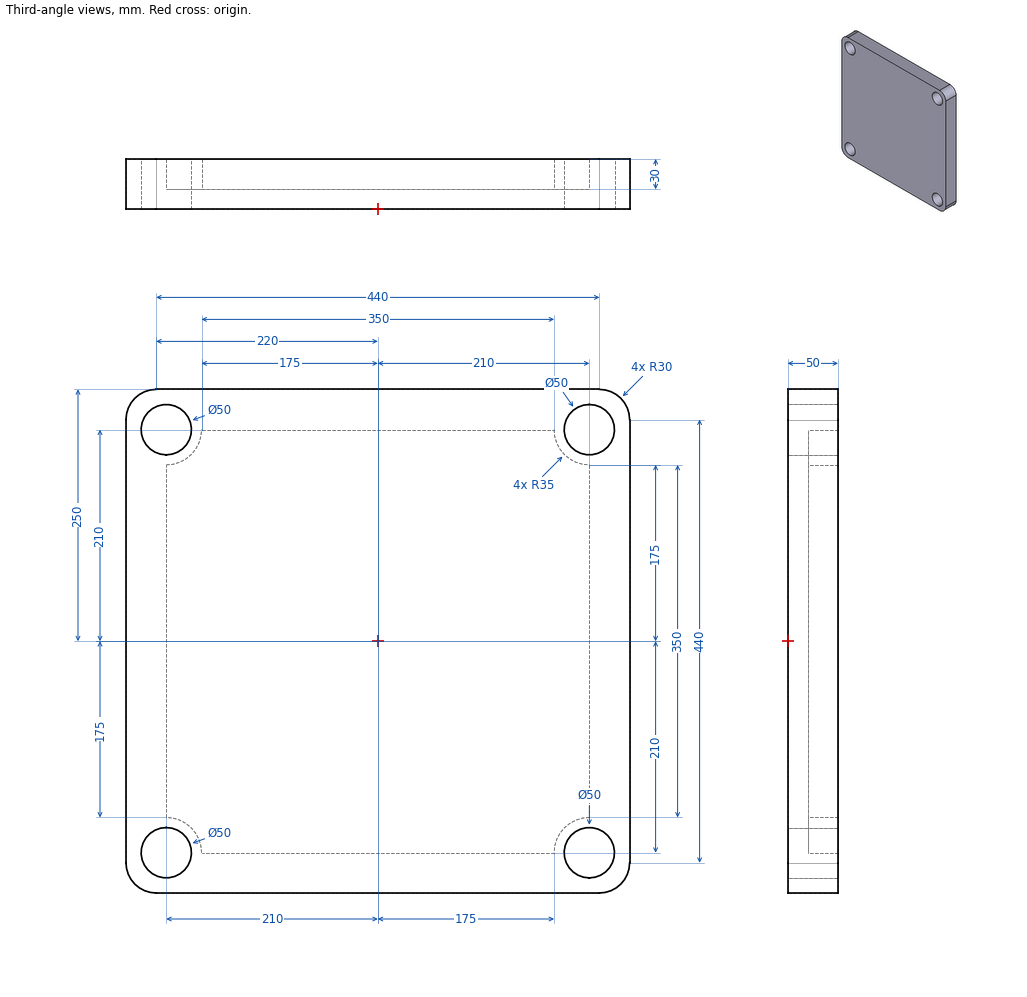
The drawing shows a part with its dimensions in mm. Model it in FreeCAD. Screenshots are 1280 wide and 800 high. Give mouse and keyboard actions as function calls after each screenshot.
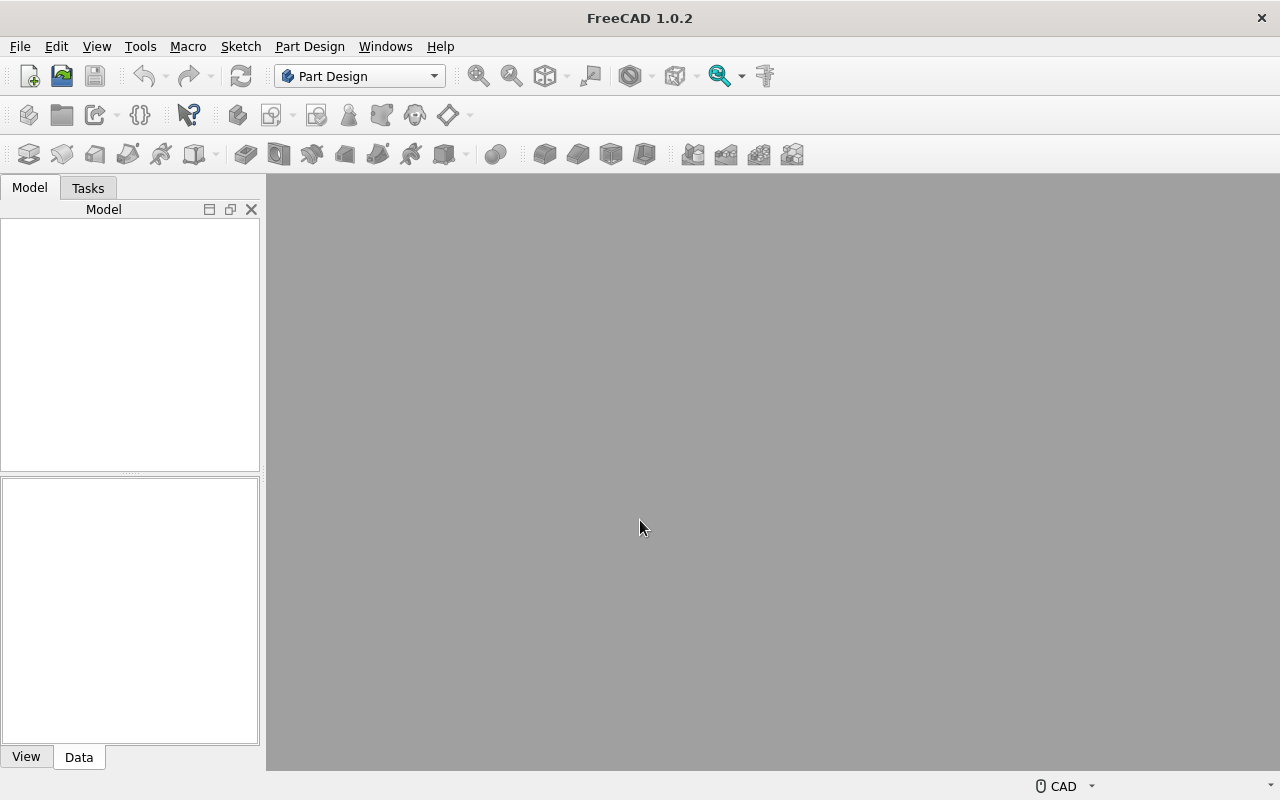
click(29, 76)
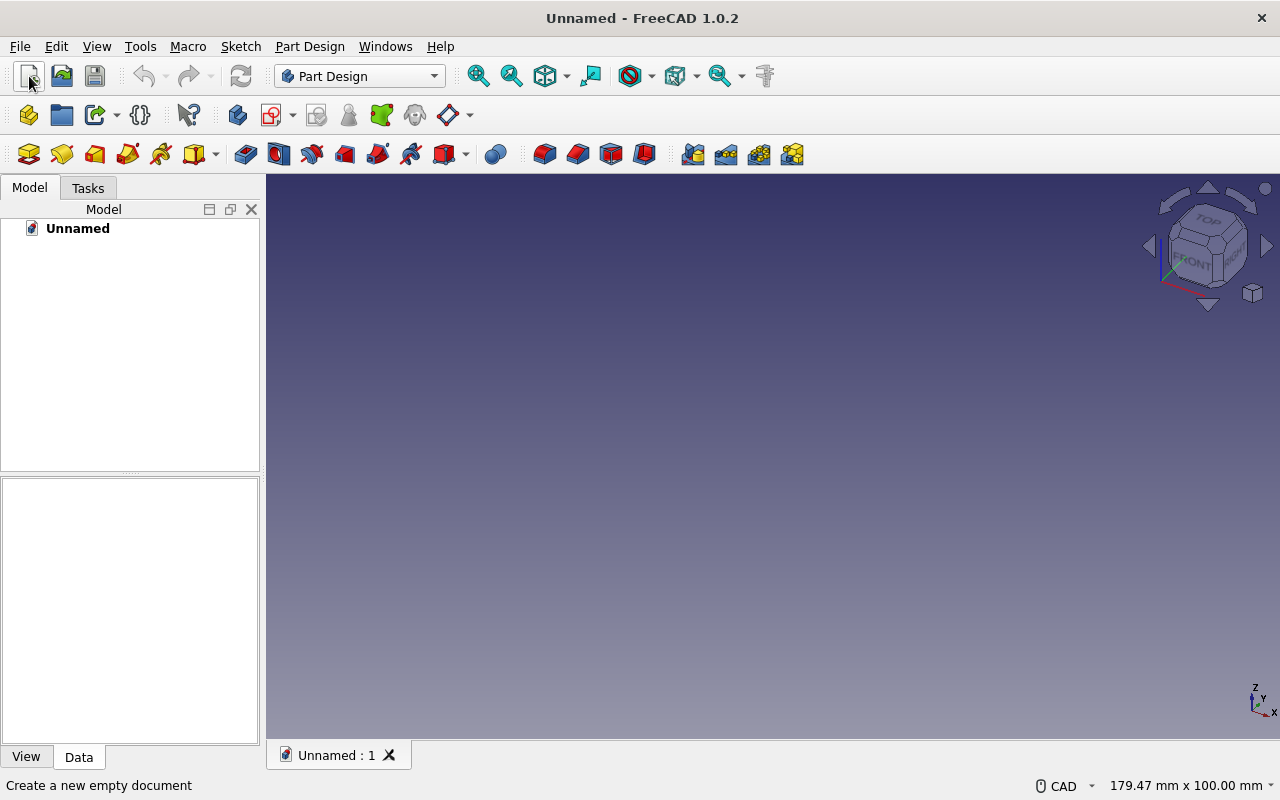
click(270, 116)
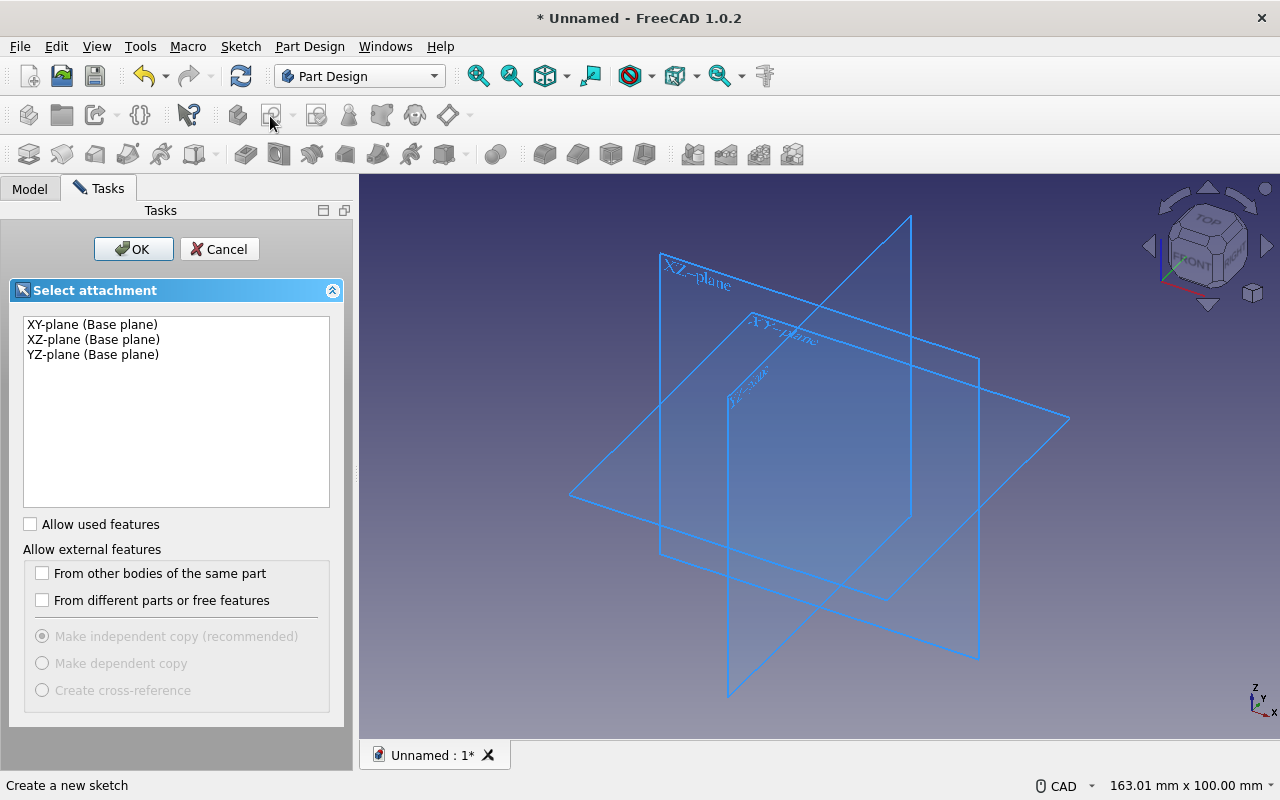
click(84, 340)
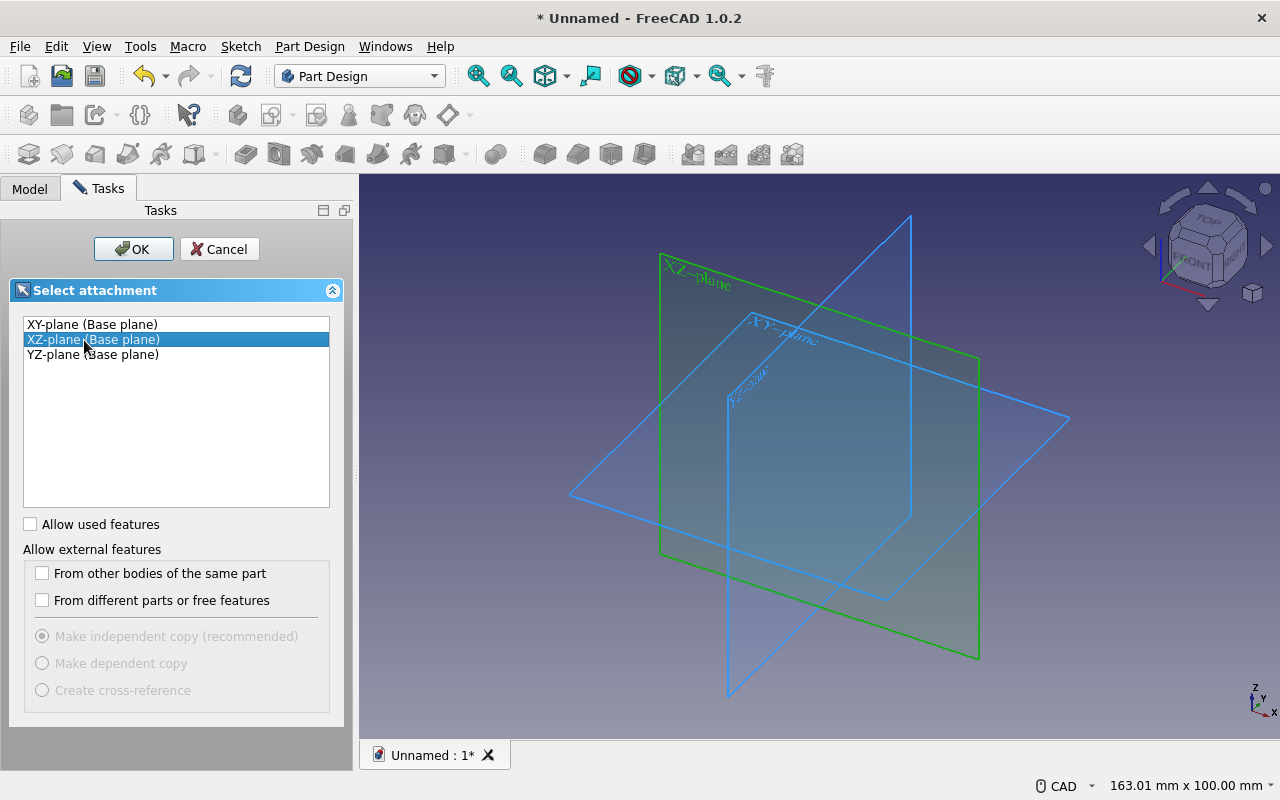
click(134, 249)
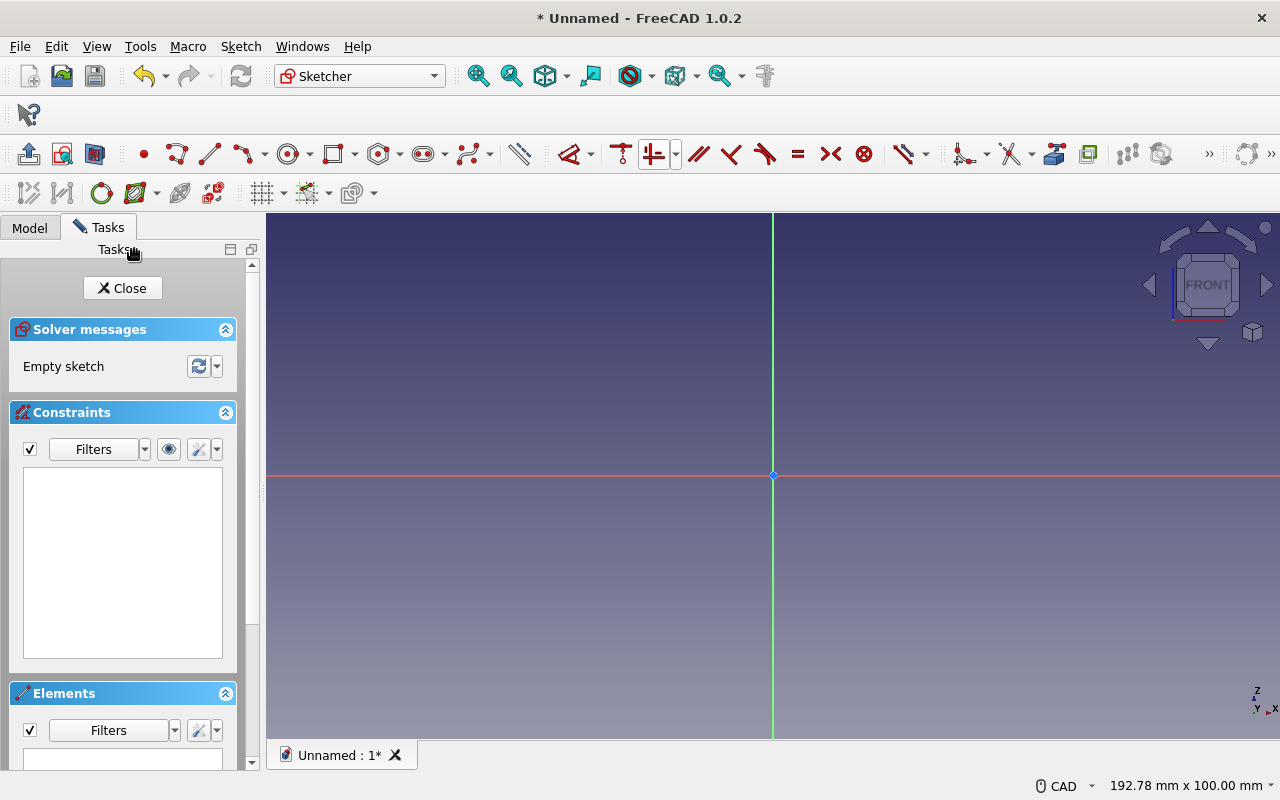
scroll(694, 476, down, 10)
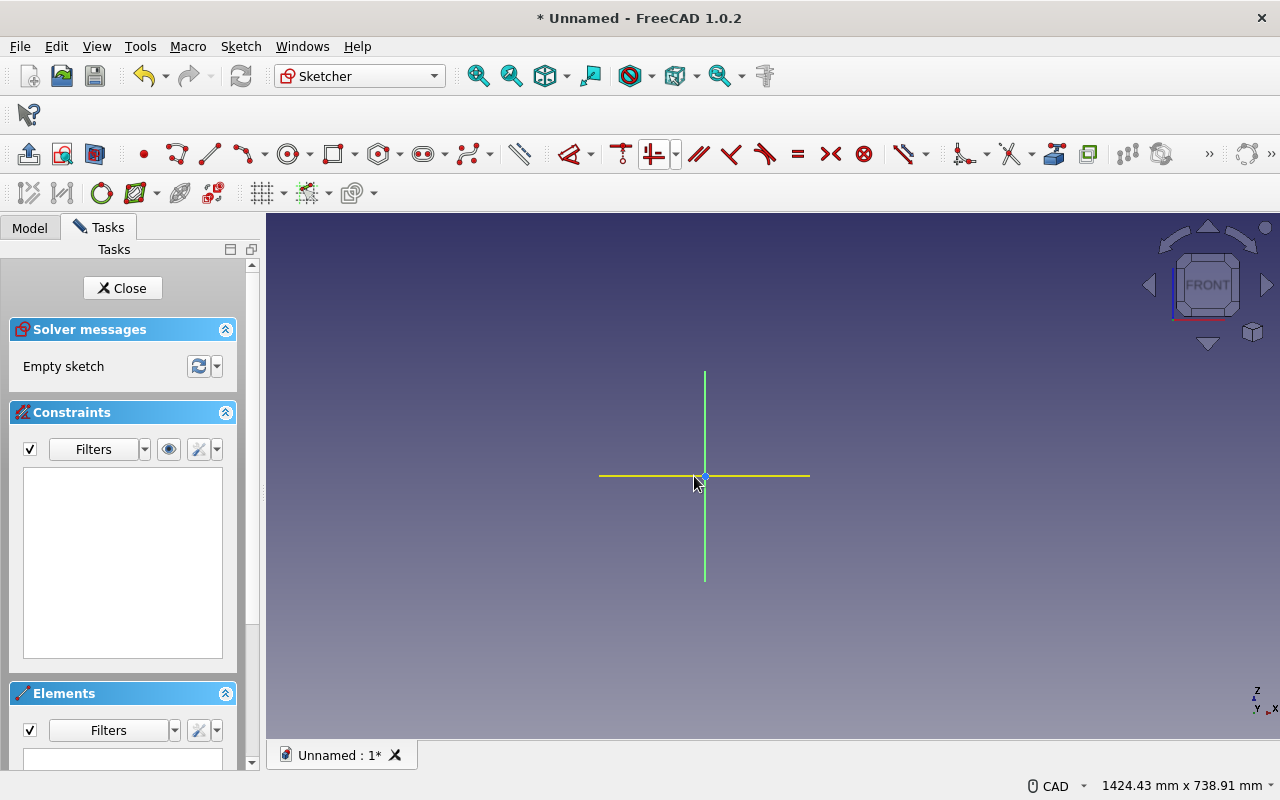
click(210, 154)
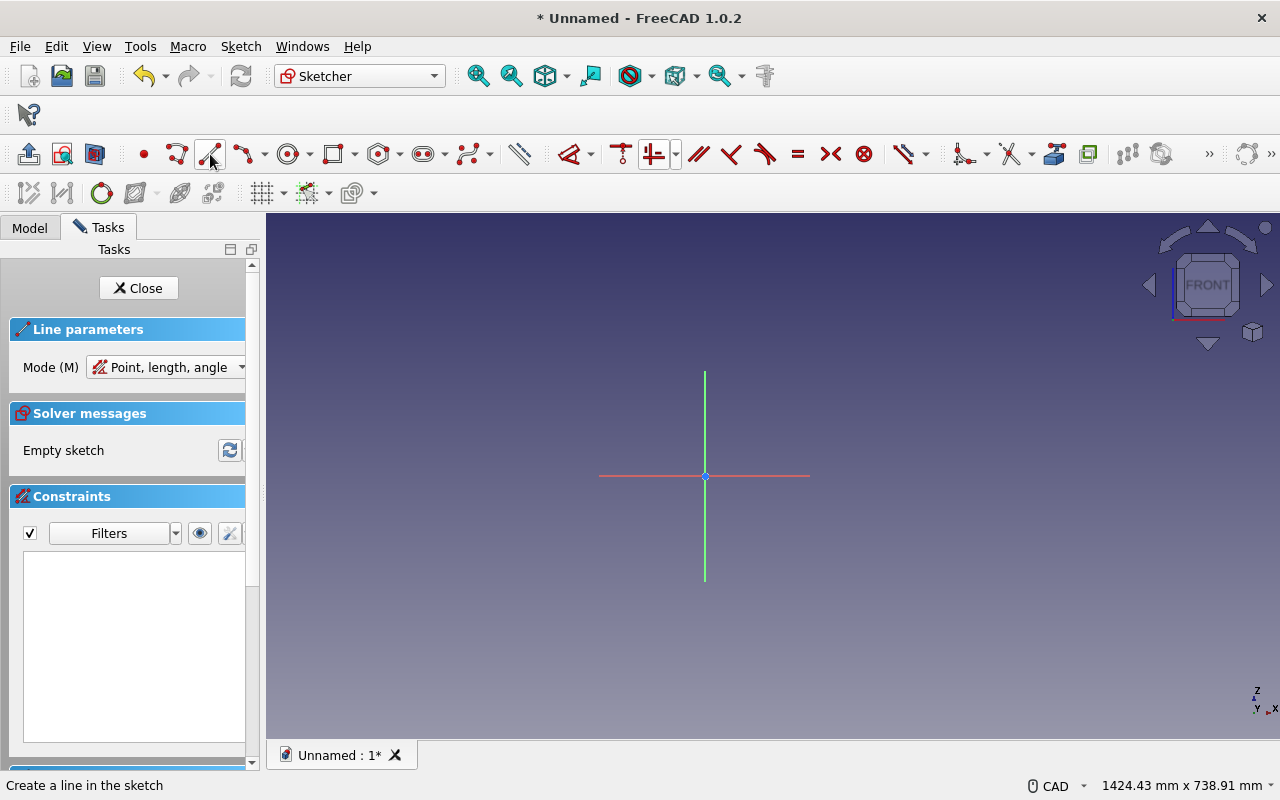
click(548, 298)
click(862, 298)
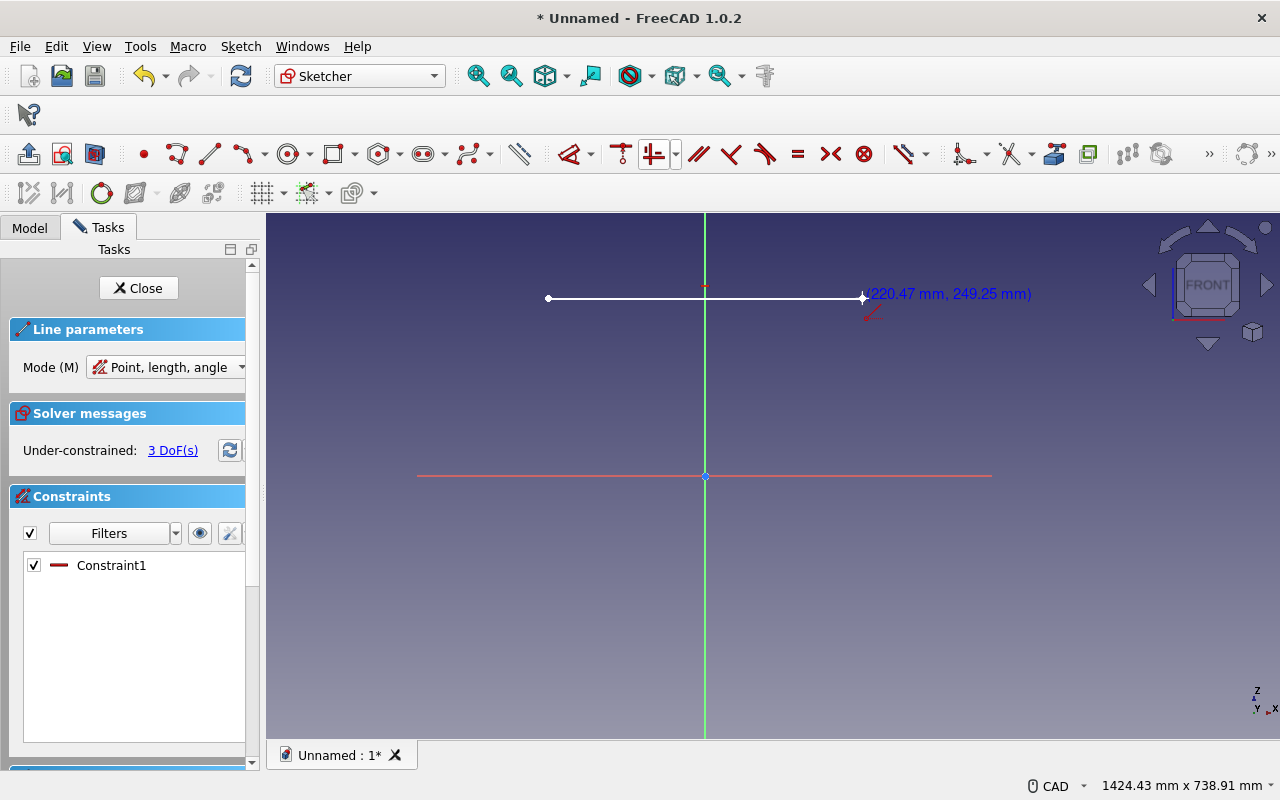
click(883, 320)
click(883, 633)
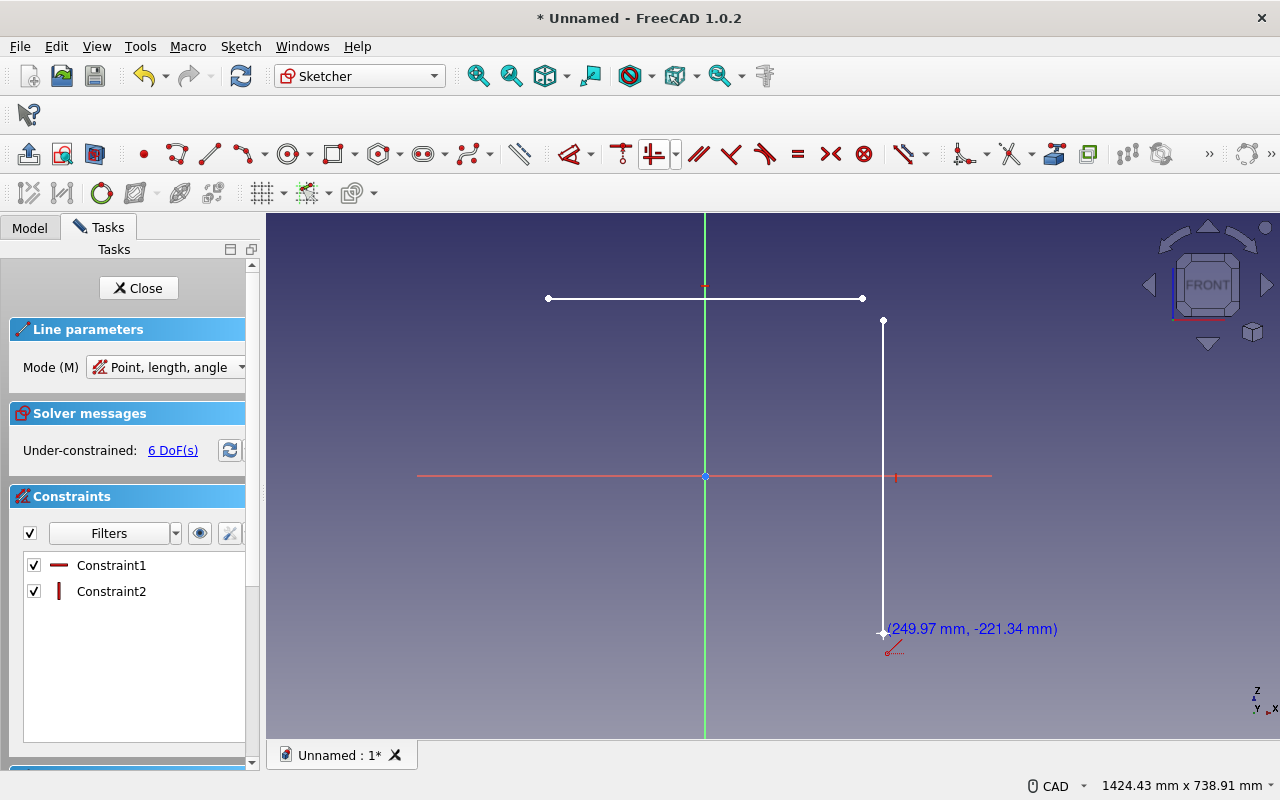
click(862, 654)
click(548, 654)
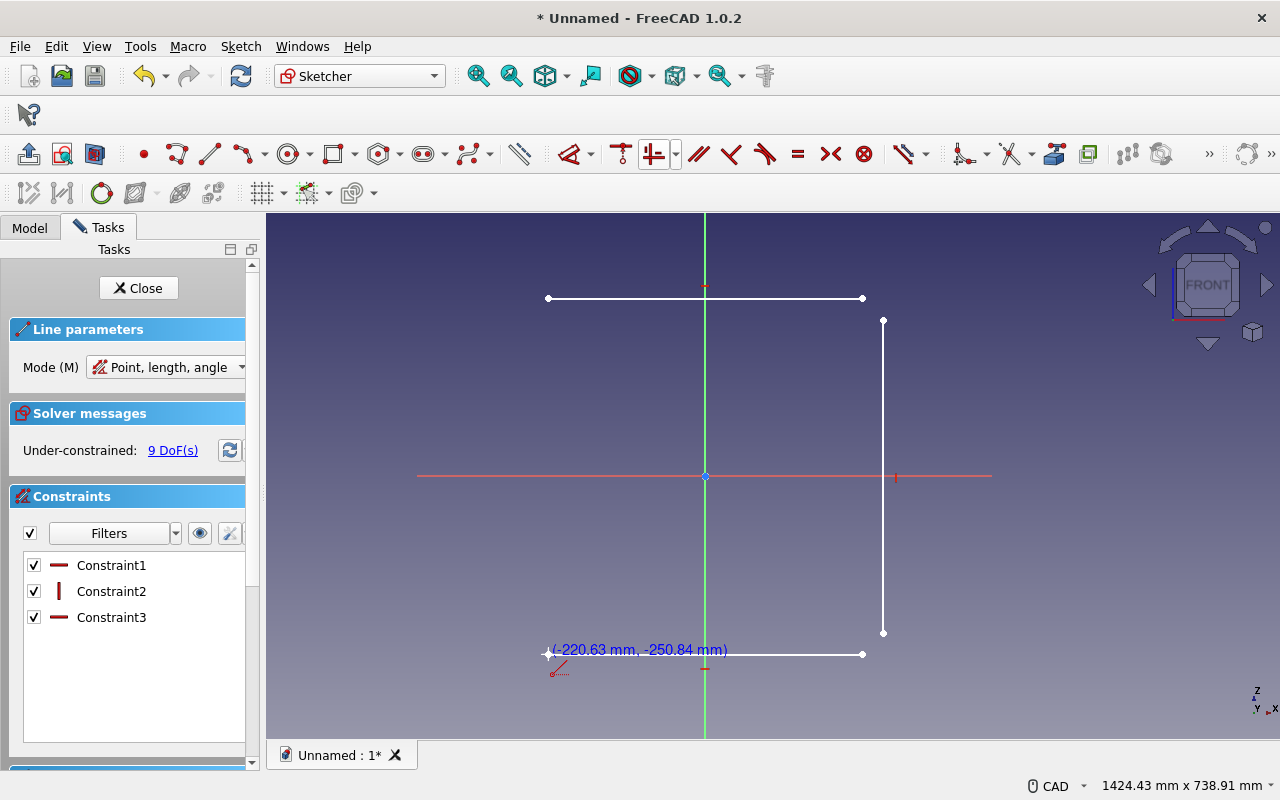
click(527, 633)
click(527, 320)